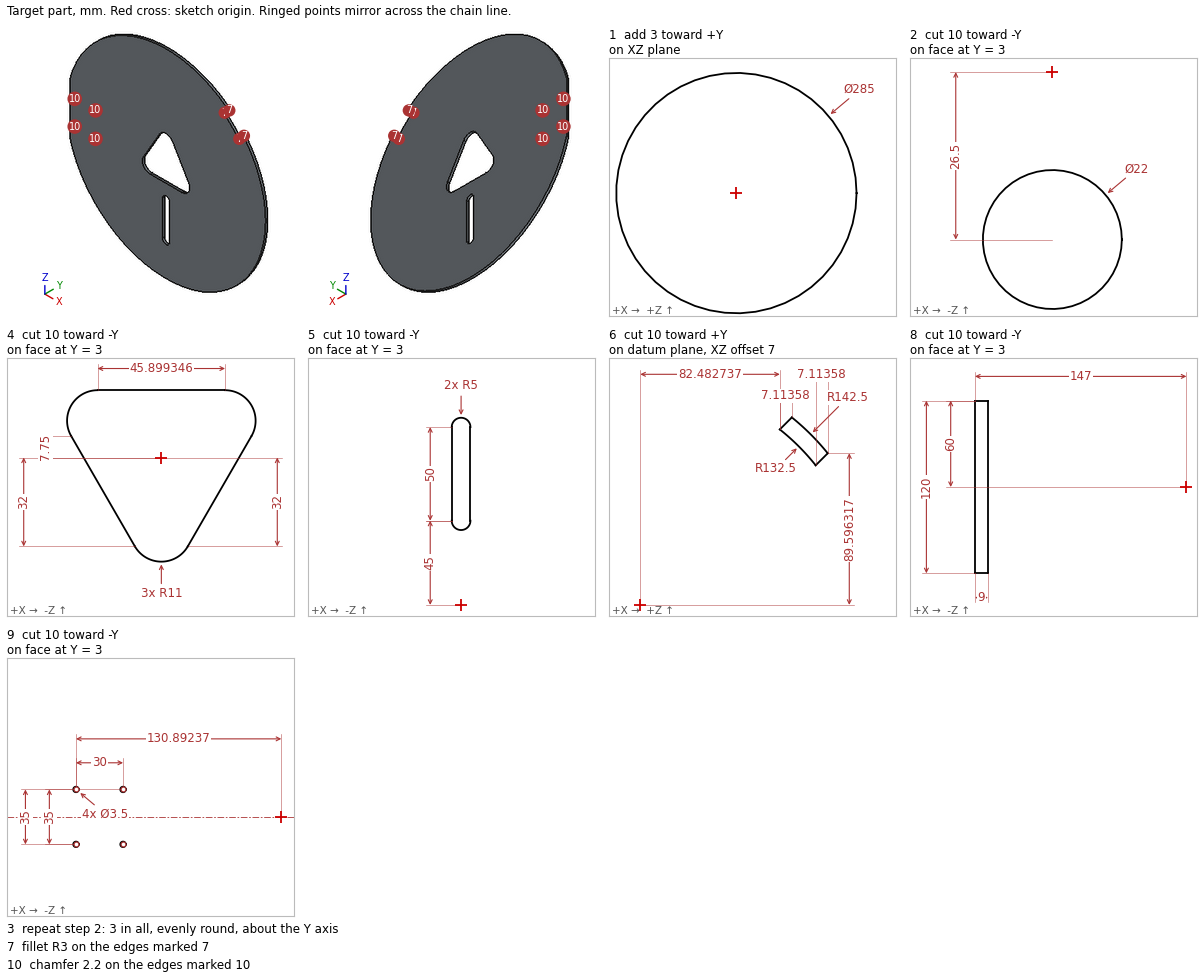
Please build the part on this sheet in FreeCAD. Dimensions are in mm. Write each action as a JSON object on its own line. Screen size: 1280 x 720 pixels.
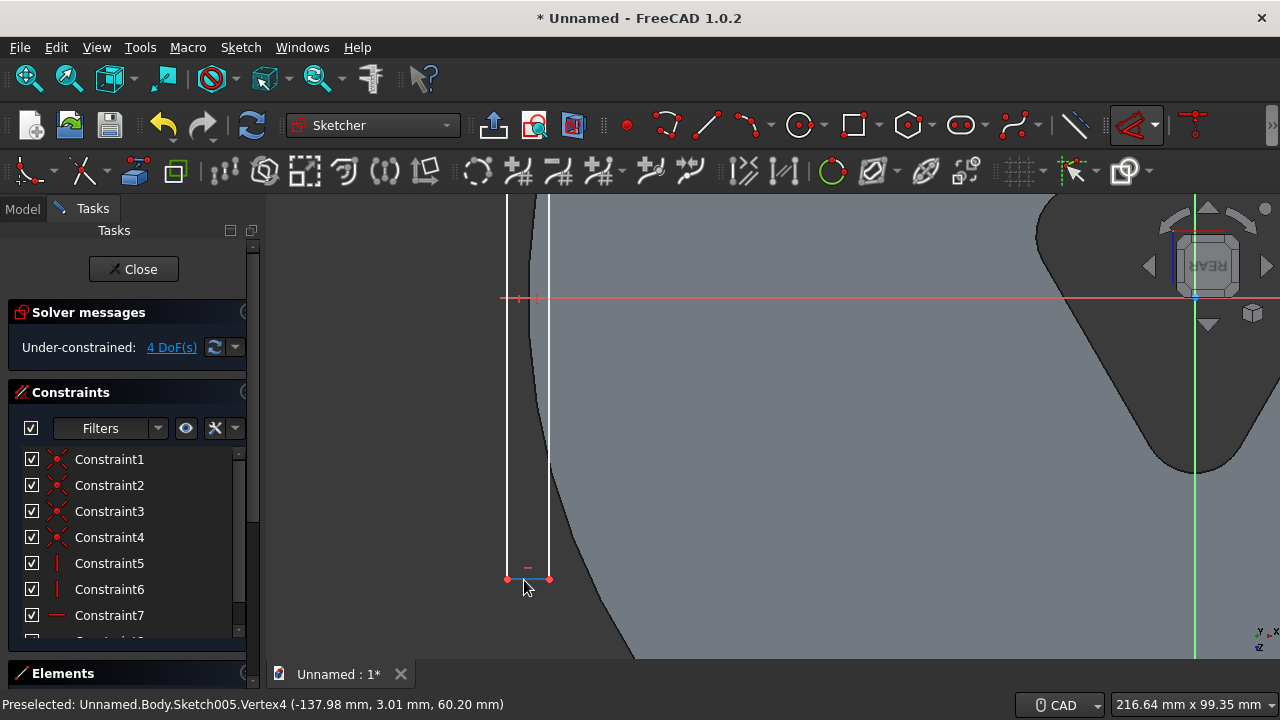
{"action": "left_click", "coordinate": [524, 579]}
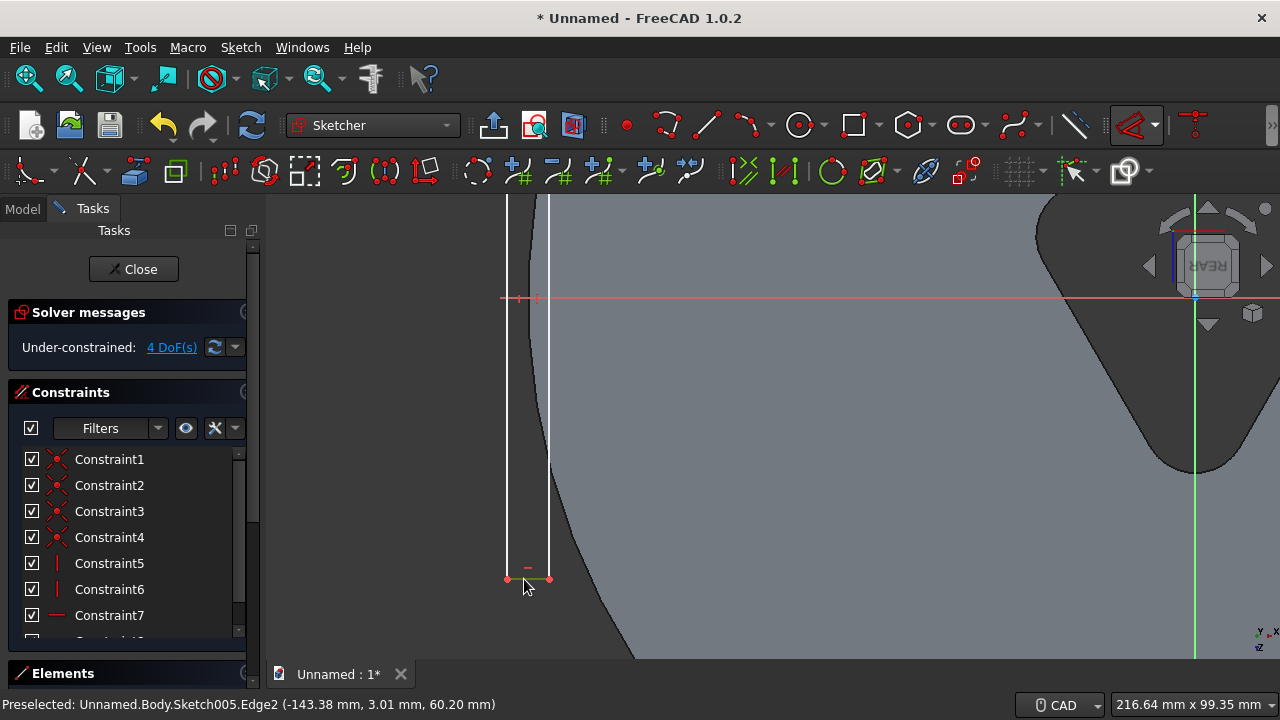
{"action": "key", "text": "l"}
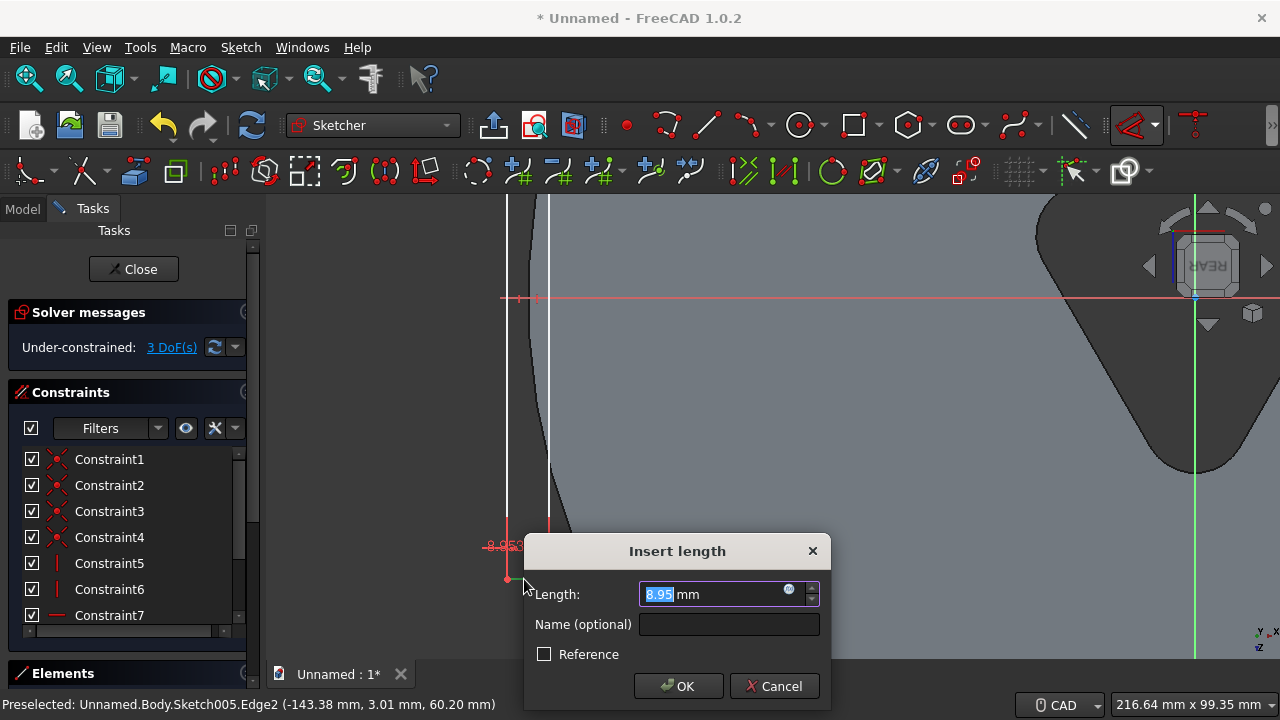
{"action": "type", "text": "9"}
{"action": "key", "text": "Return"}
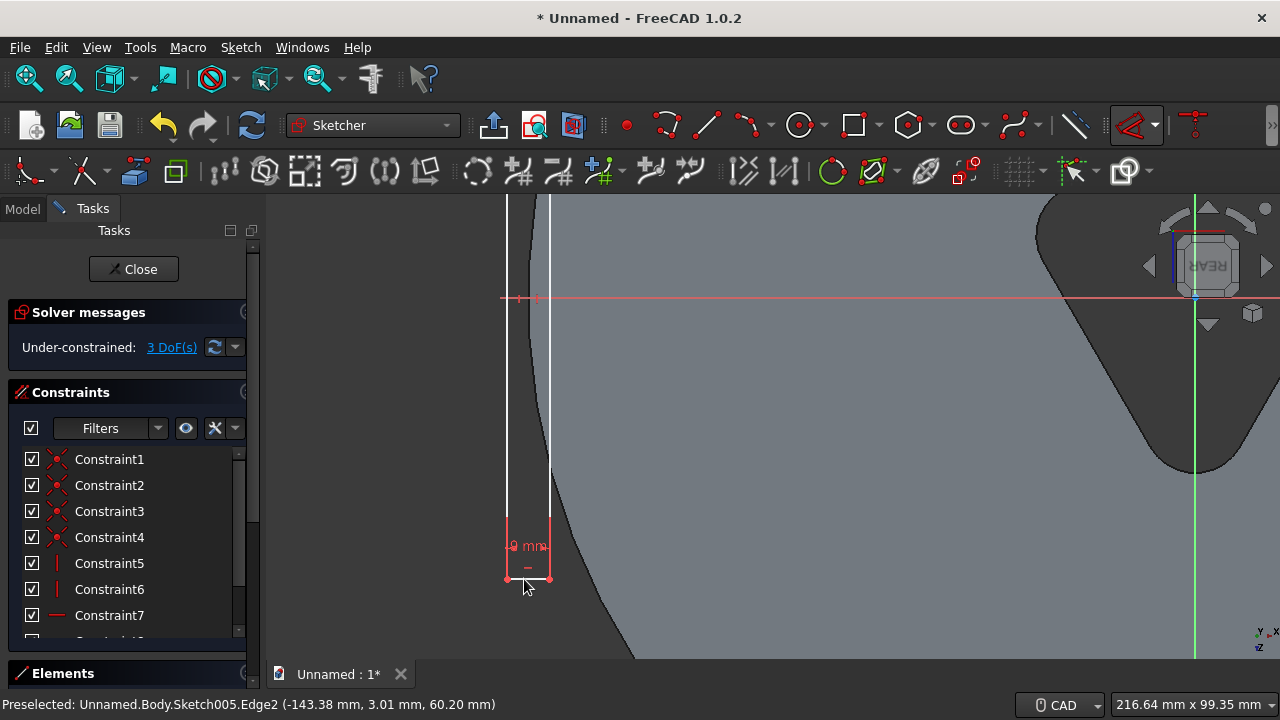
{"action": "left_click", "coordinate": [507, 411]}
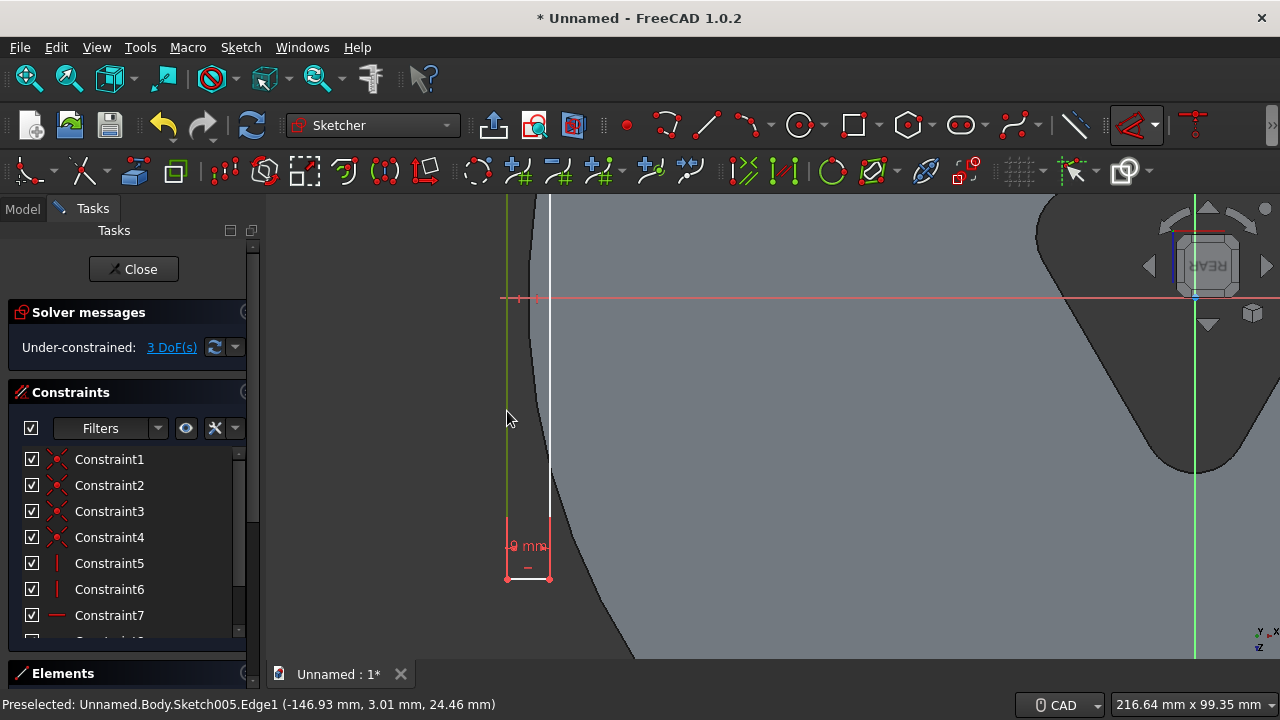
{"action": "key", "text": "i"}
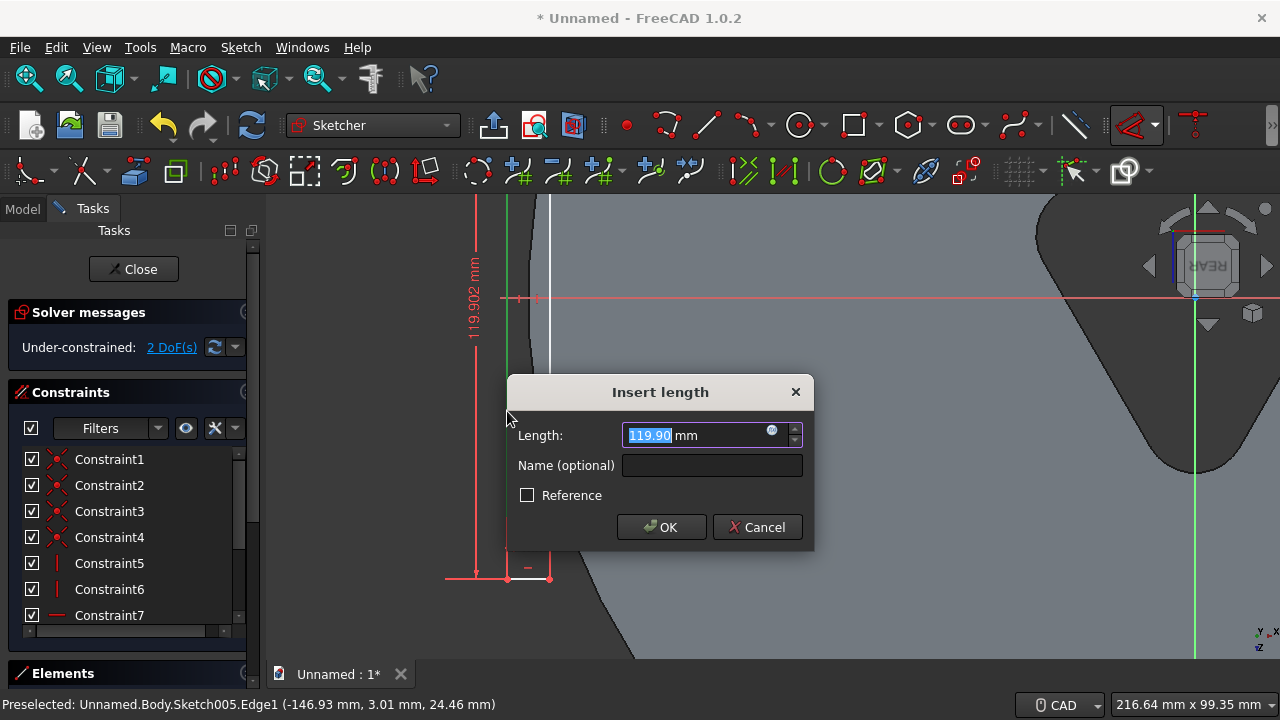
{"action": "type", "text": "120"}
{"action": "key", "text": "Return"}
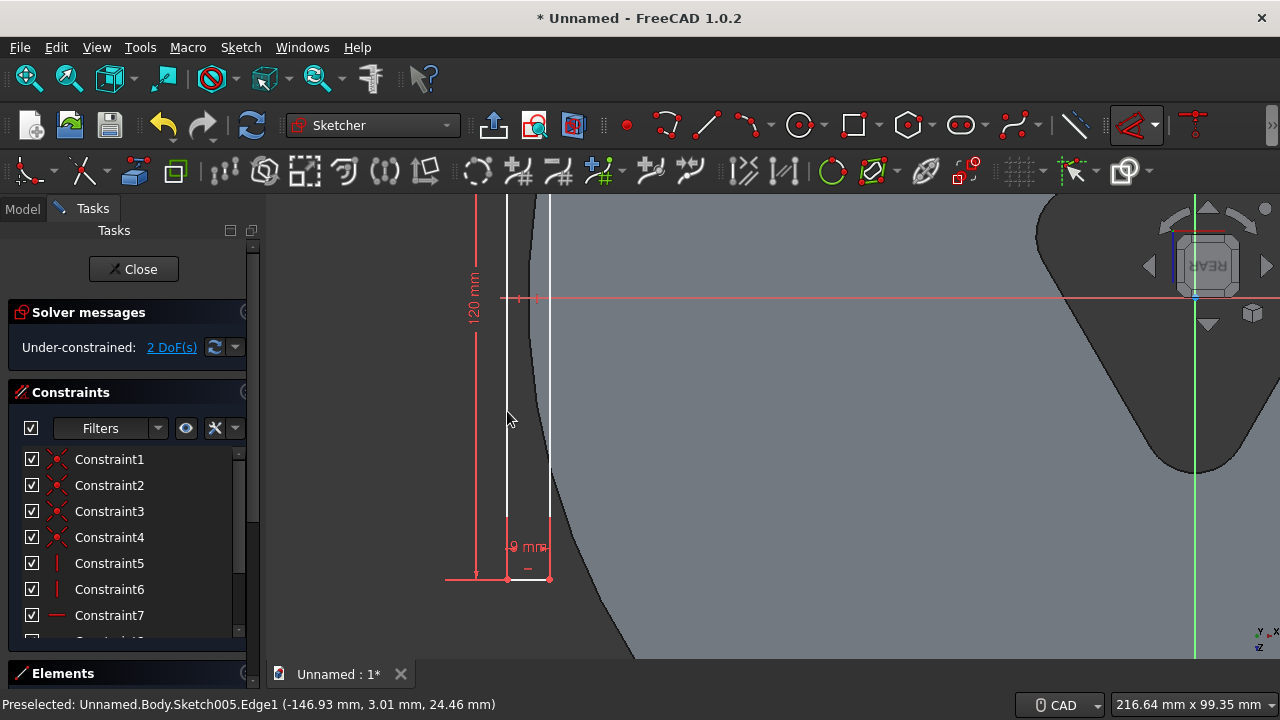
{"action": "scroll", "coordinate": [526, 583], "scroll_direction": "down", "scroll_amount": 3}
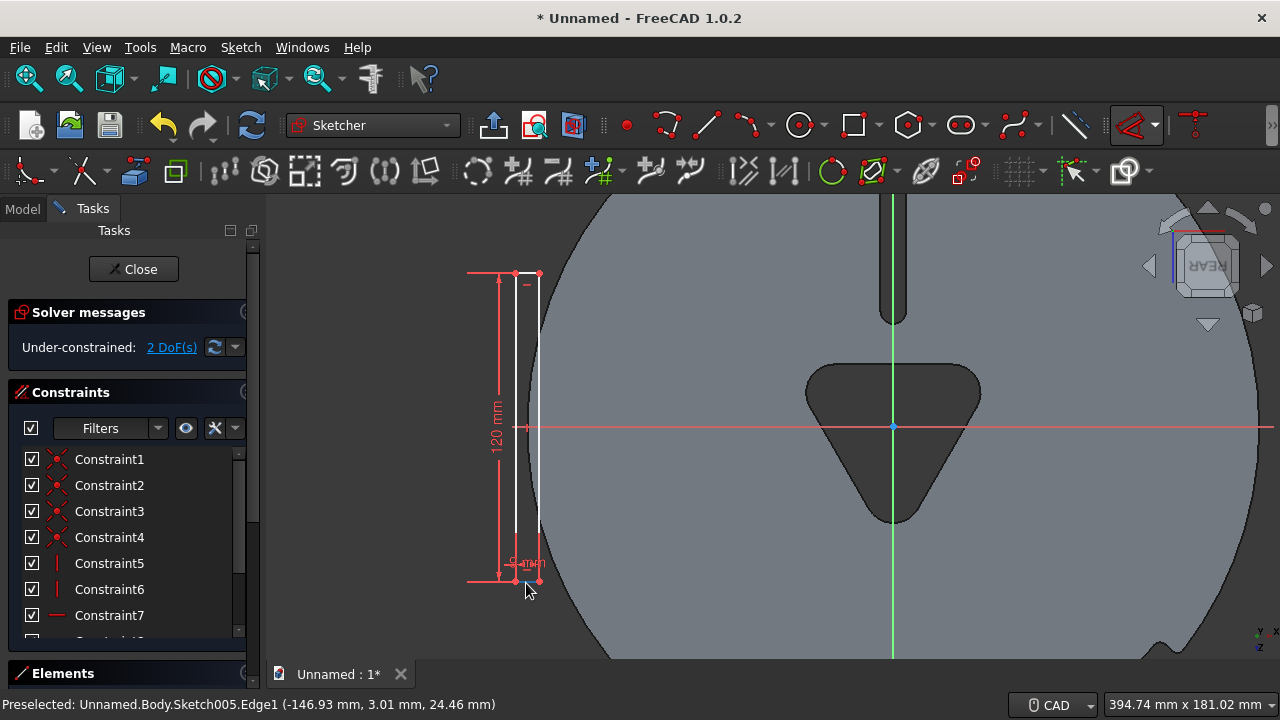
{"action": "left_click", "coordinate": [516, 273]}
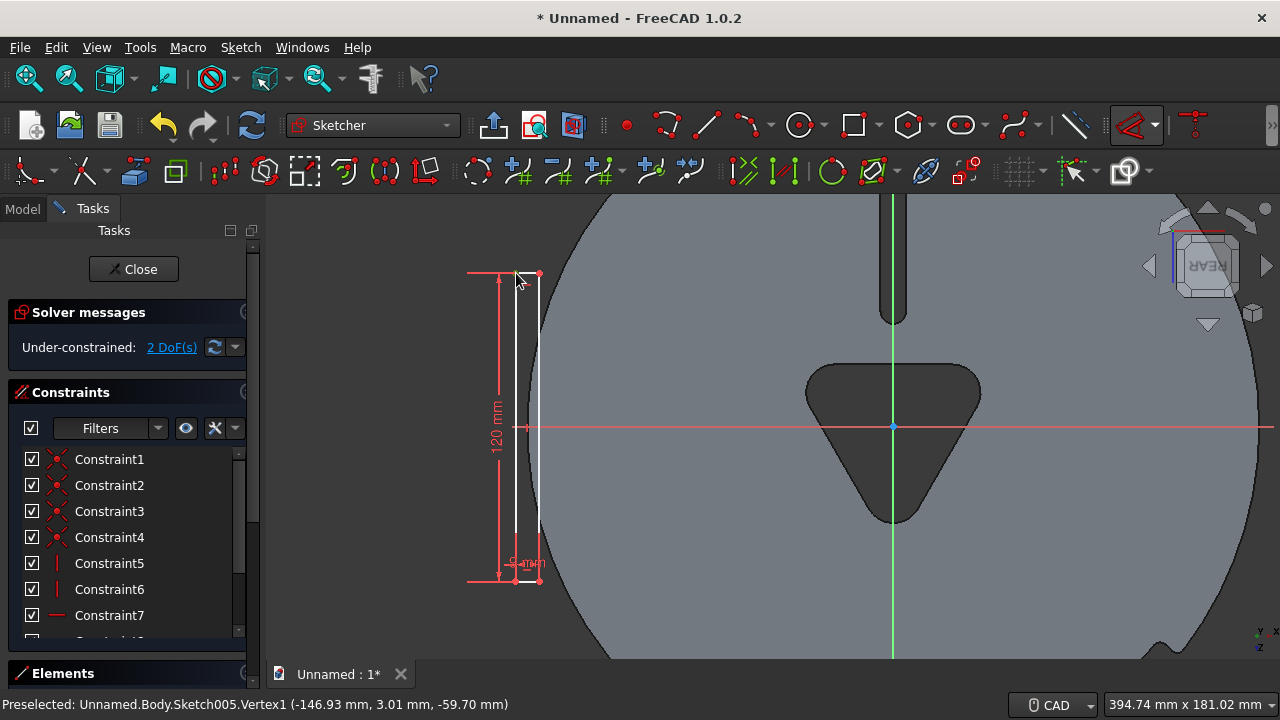
{"action": "left_click", "coordinate": [1158, 126]}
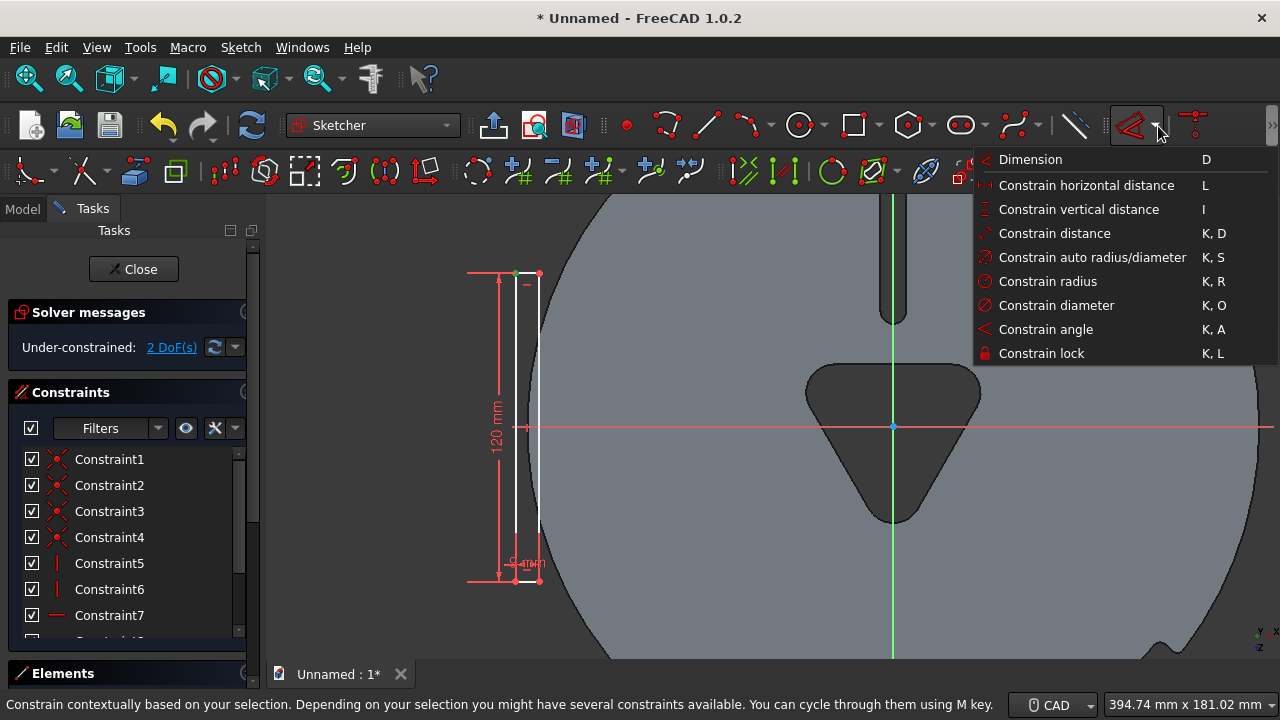
{"action": "left_click", "coordinate": [1126, 209]}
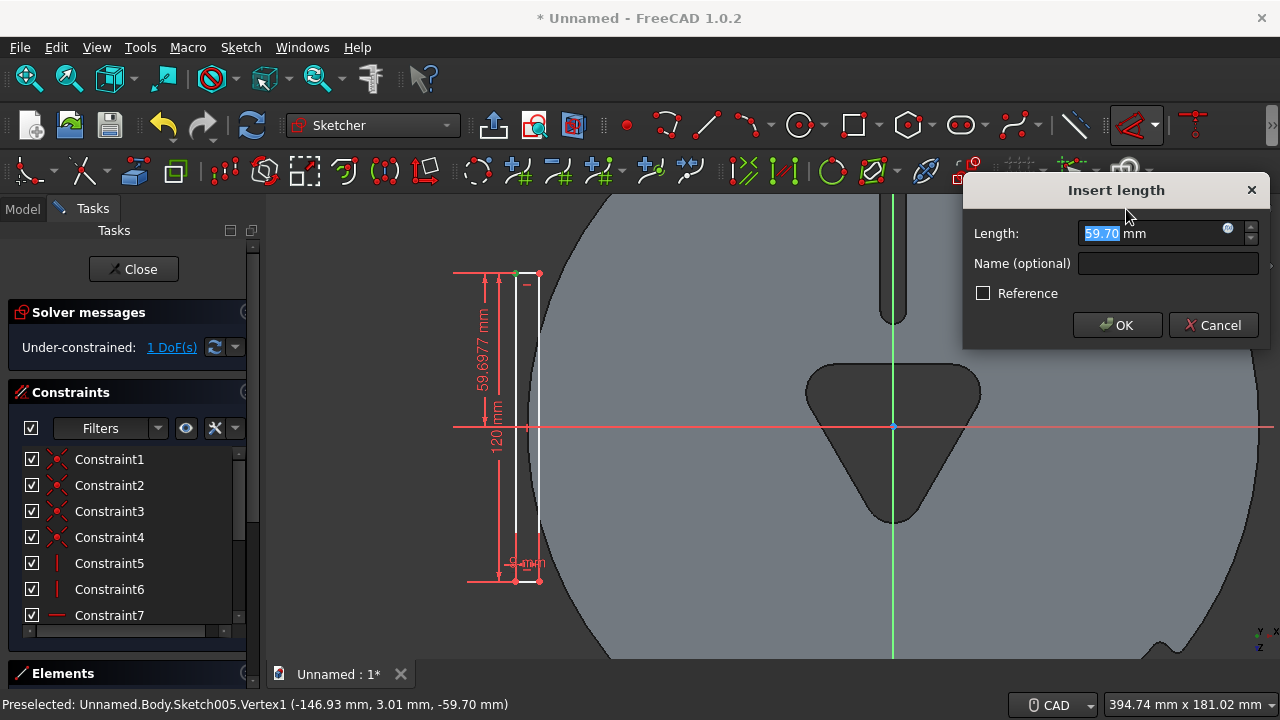
{"action": "type", "text": "60"}
{"action": "key", "text": "Return"}